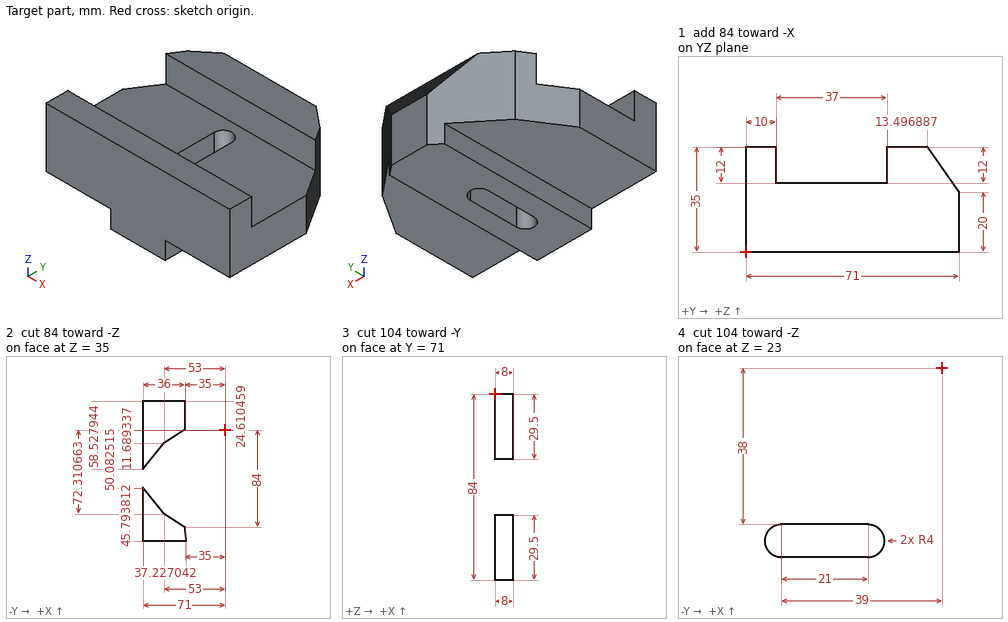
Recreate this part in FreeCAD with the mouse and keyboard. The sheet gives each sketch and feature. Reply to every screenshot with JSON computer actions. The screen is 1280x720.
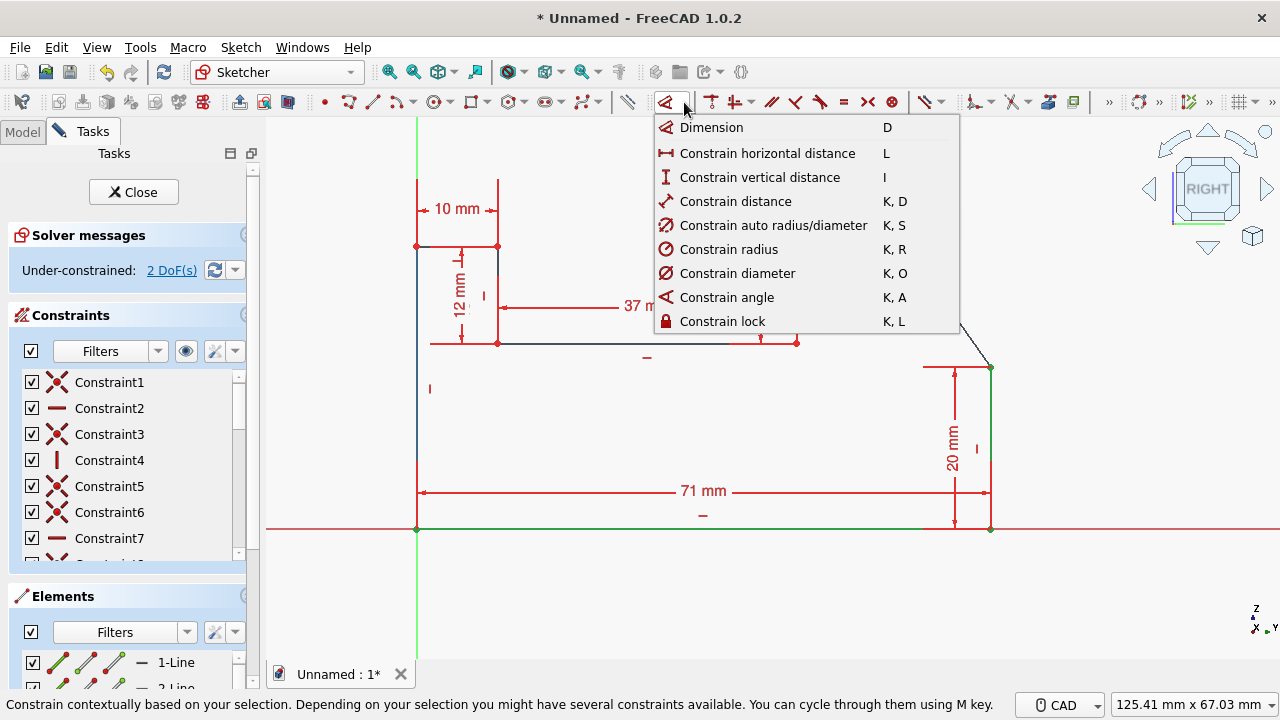
{"action": "left_click", "coordinate": [807, 177]}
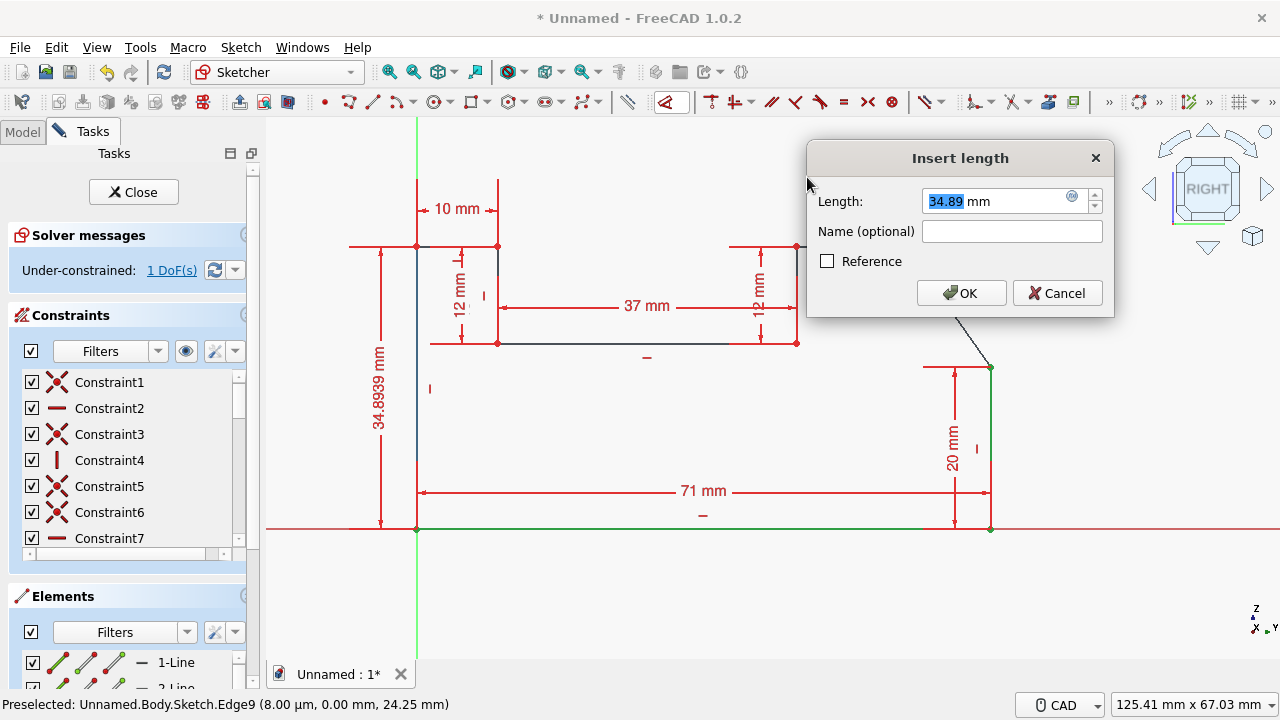
{"action": "type", "text": "35"}
{"action": "key", "text": "Return"}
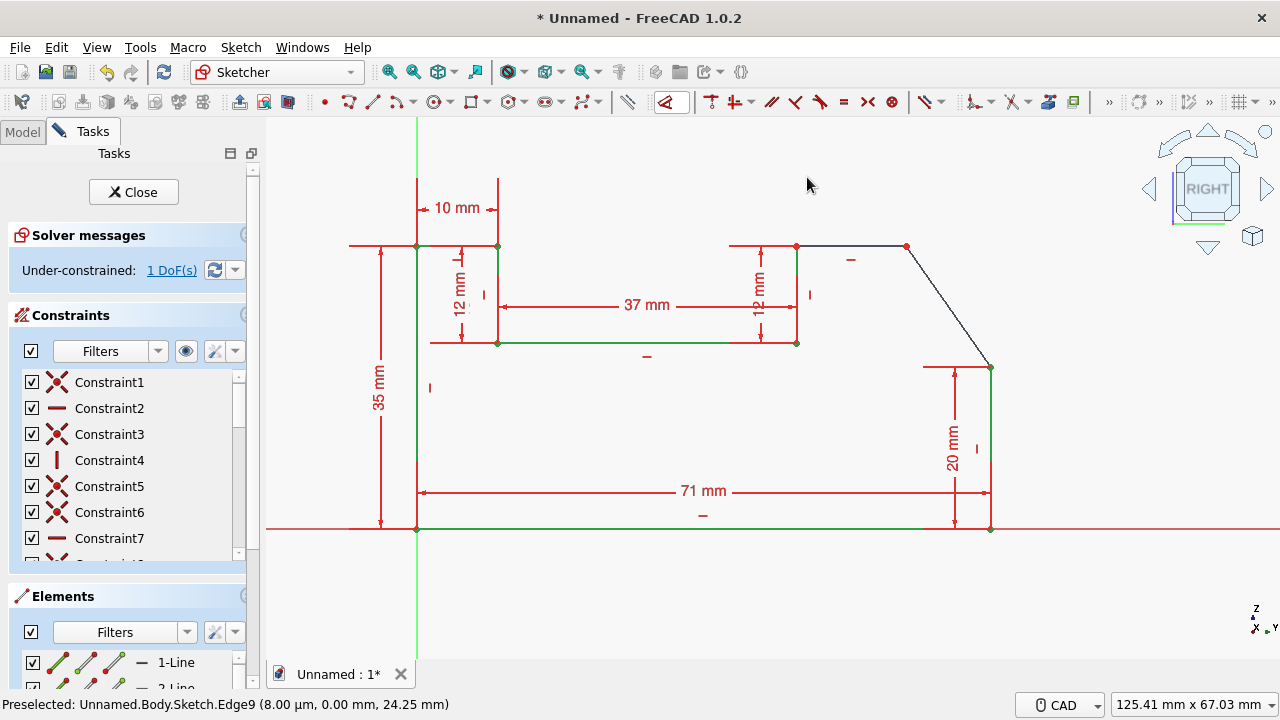
{"action": "left_click", "coordinate": [873, 246]}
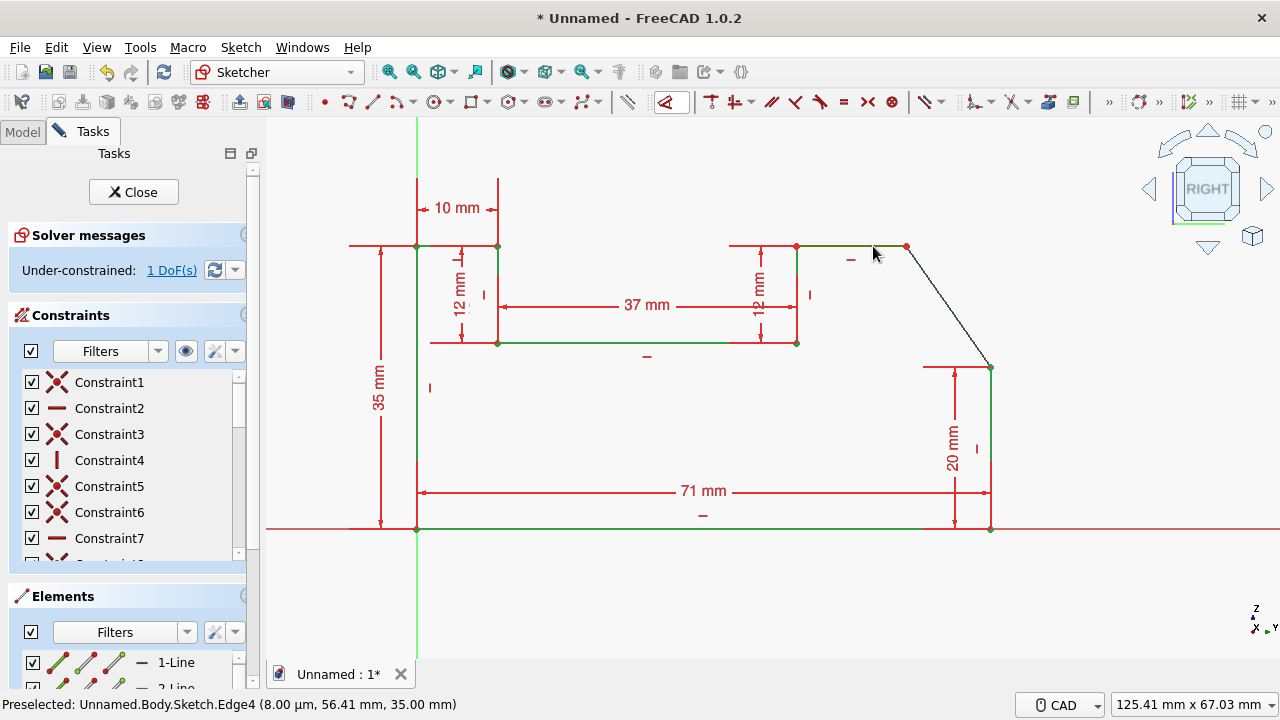
{"action": "left_click", "coordinate": [684, 102]}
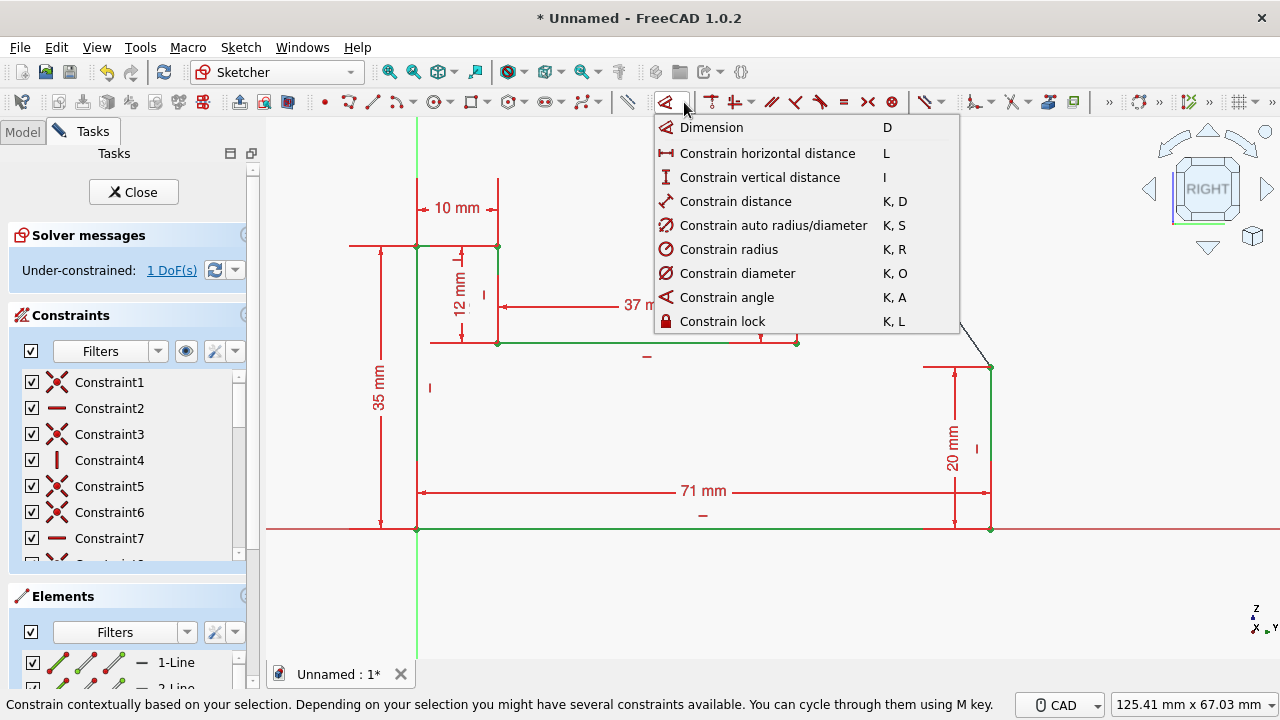
{"action": "left_click", "coordinate": [807, 153]}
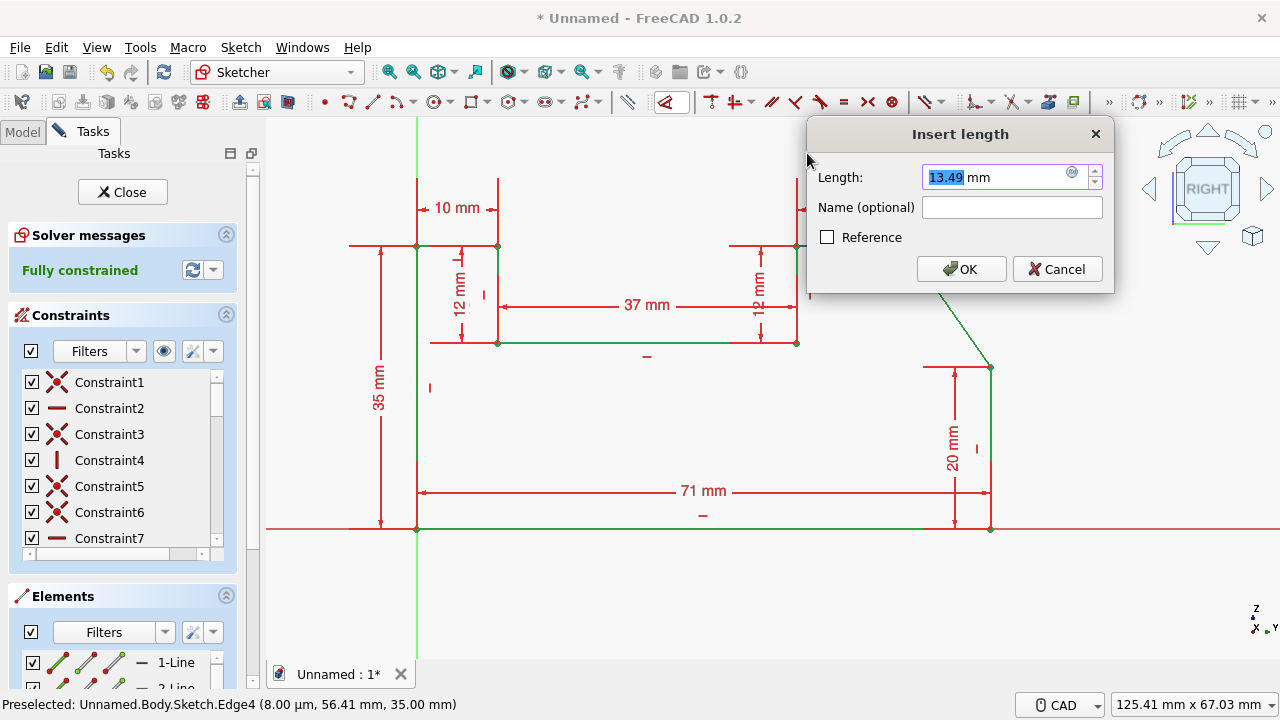
{"action": "type", "text": "13.496887"}
{"action": "key", "text": "Return"}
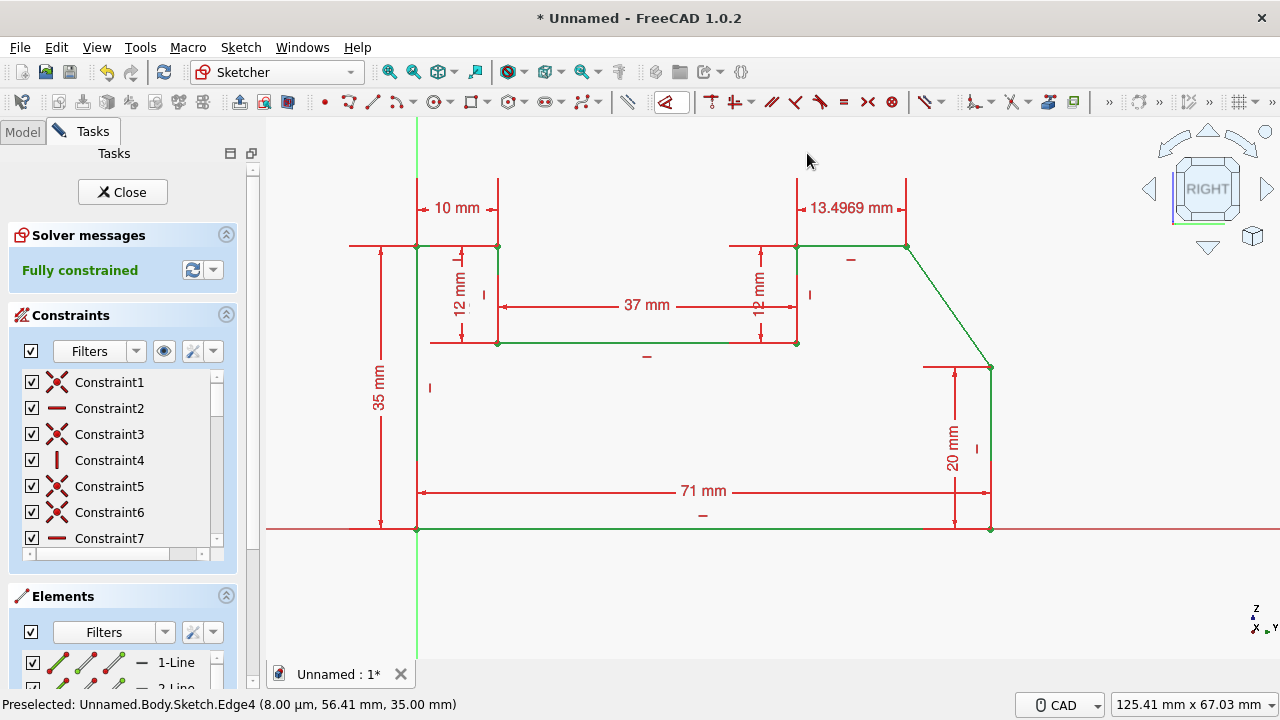
{"action": "left_click", "coordinate": [123, 192]}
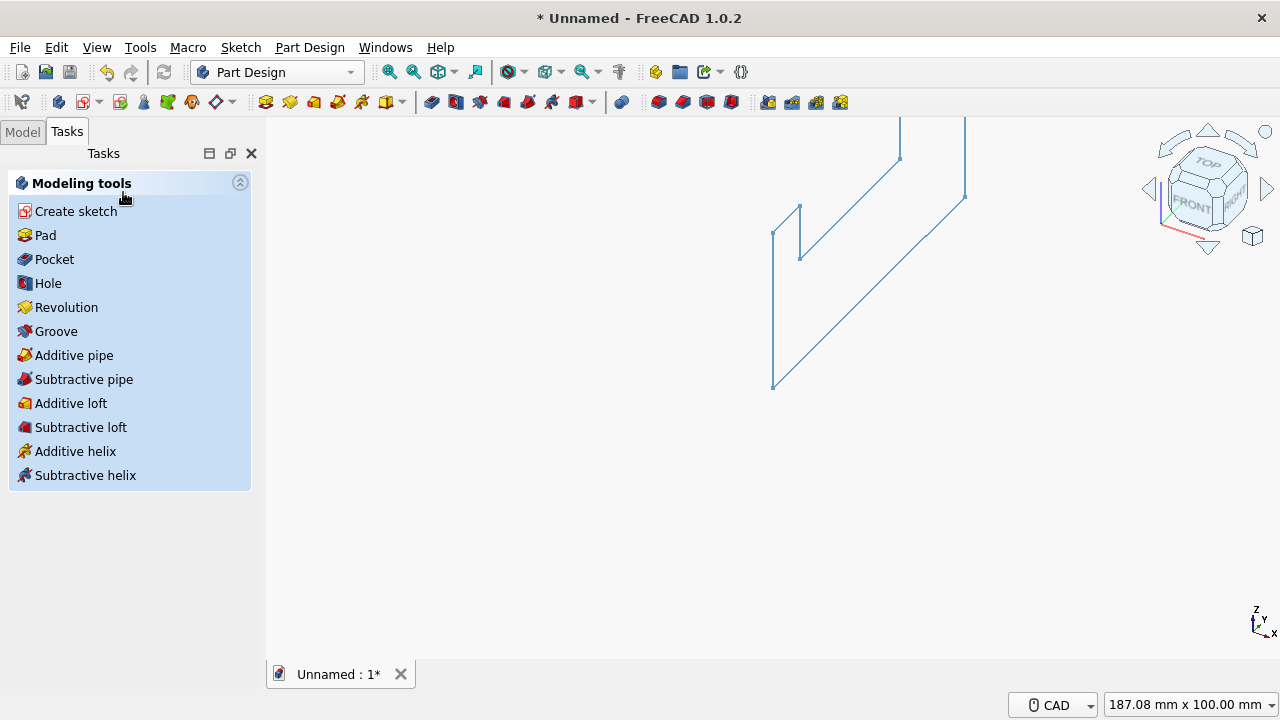
{"action": "left_click", "coordinate": [266, 102]}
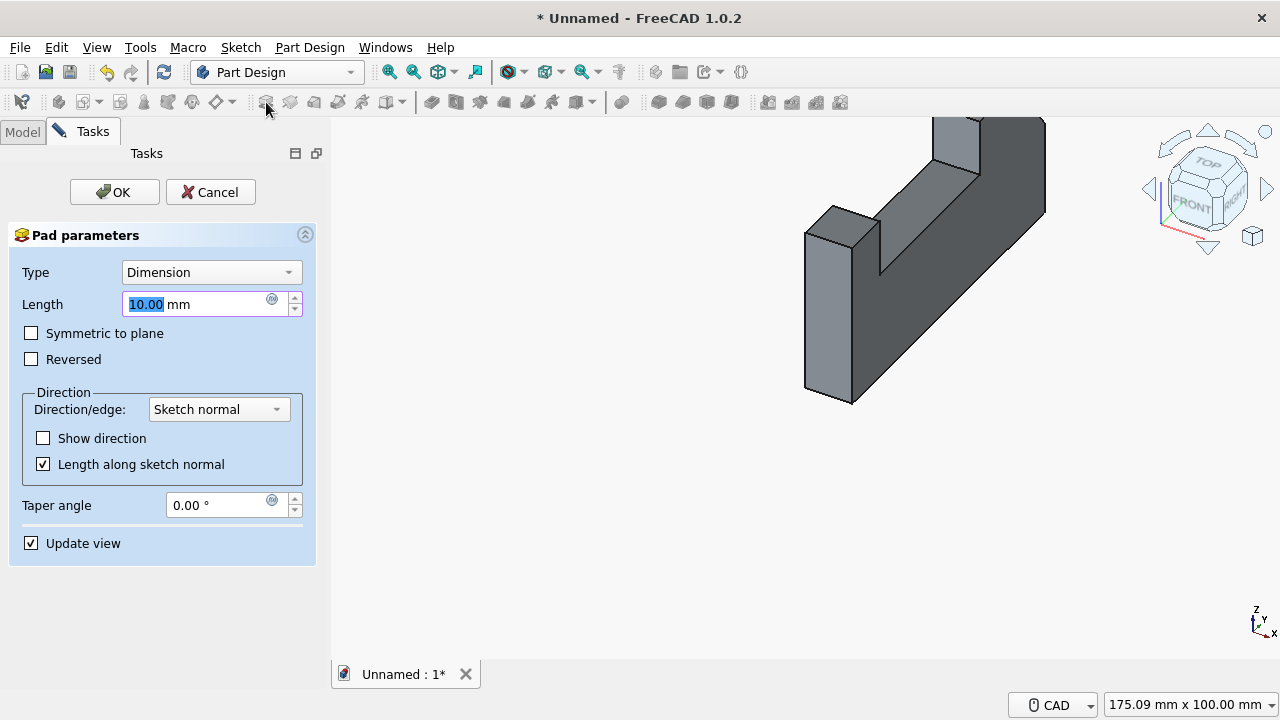
{"action": "type", "text": "84"}
{"action": "key", "text": "Tab"}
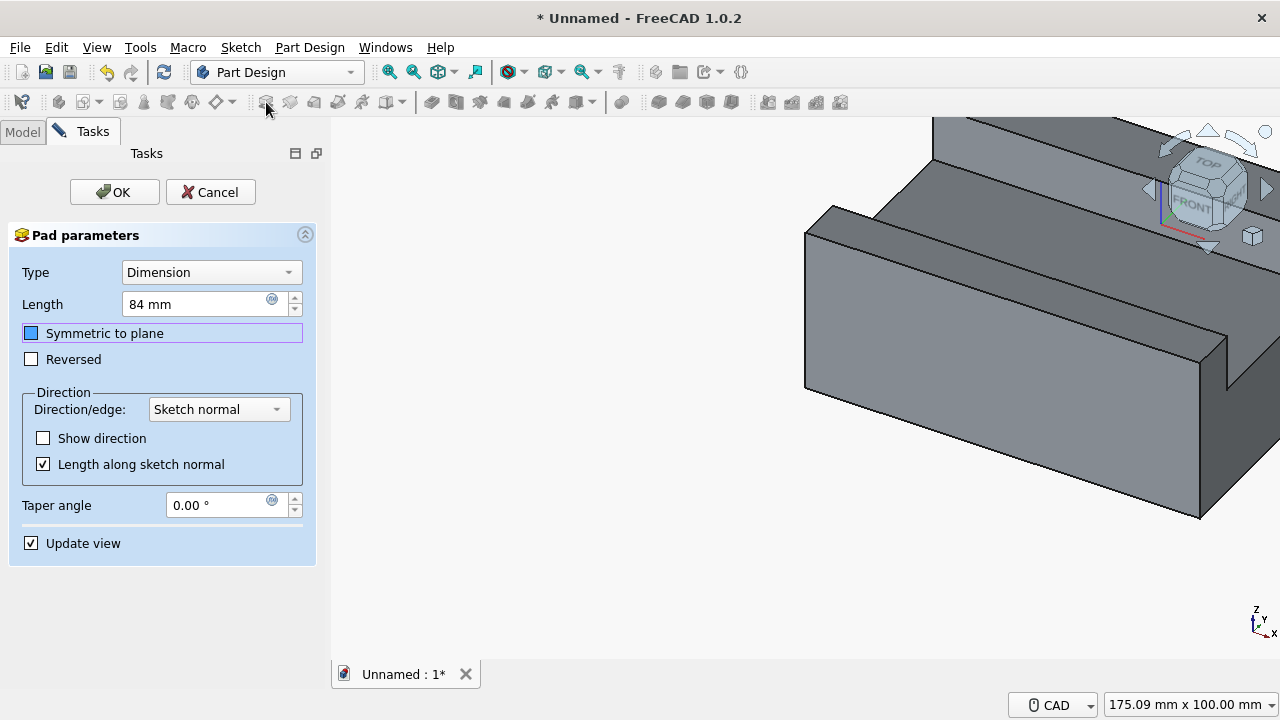
{"action": "left_click", "coordinate": [30, 359]}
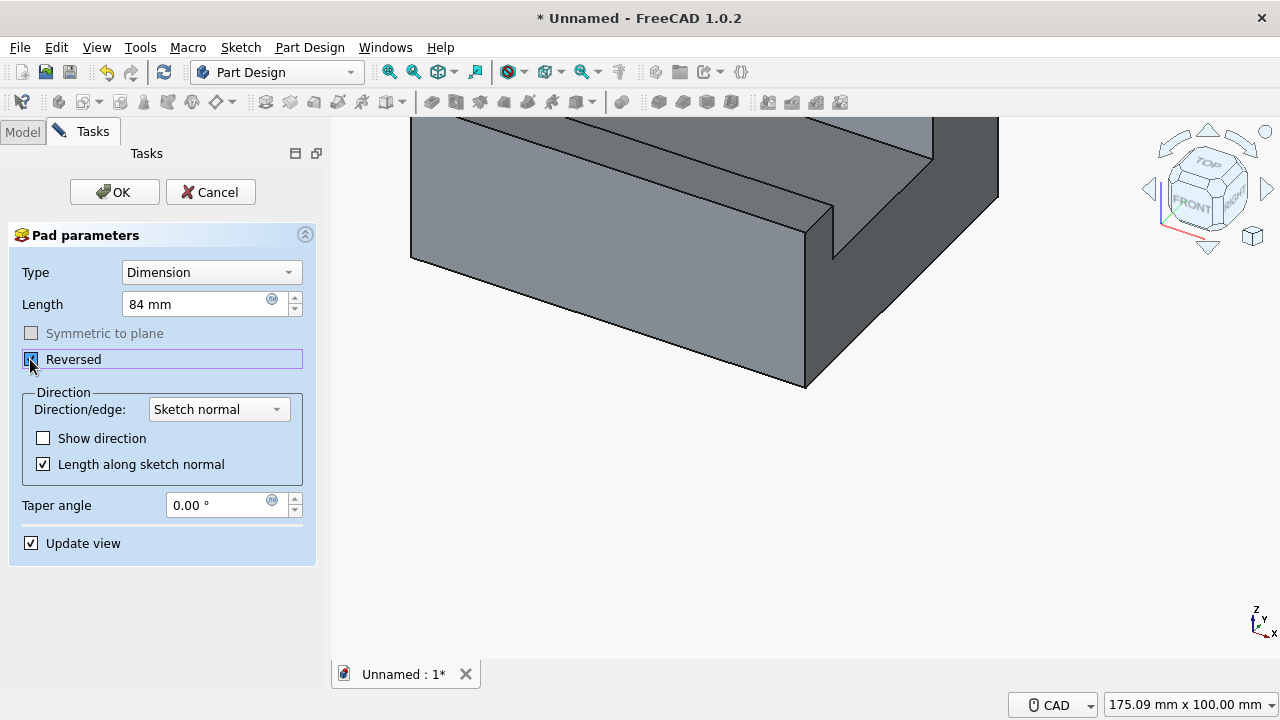
{"action": "left_click", "coordinate": [115, 192]}